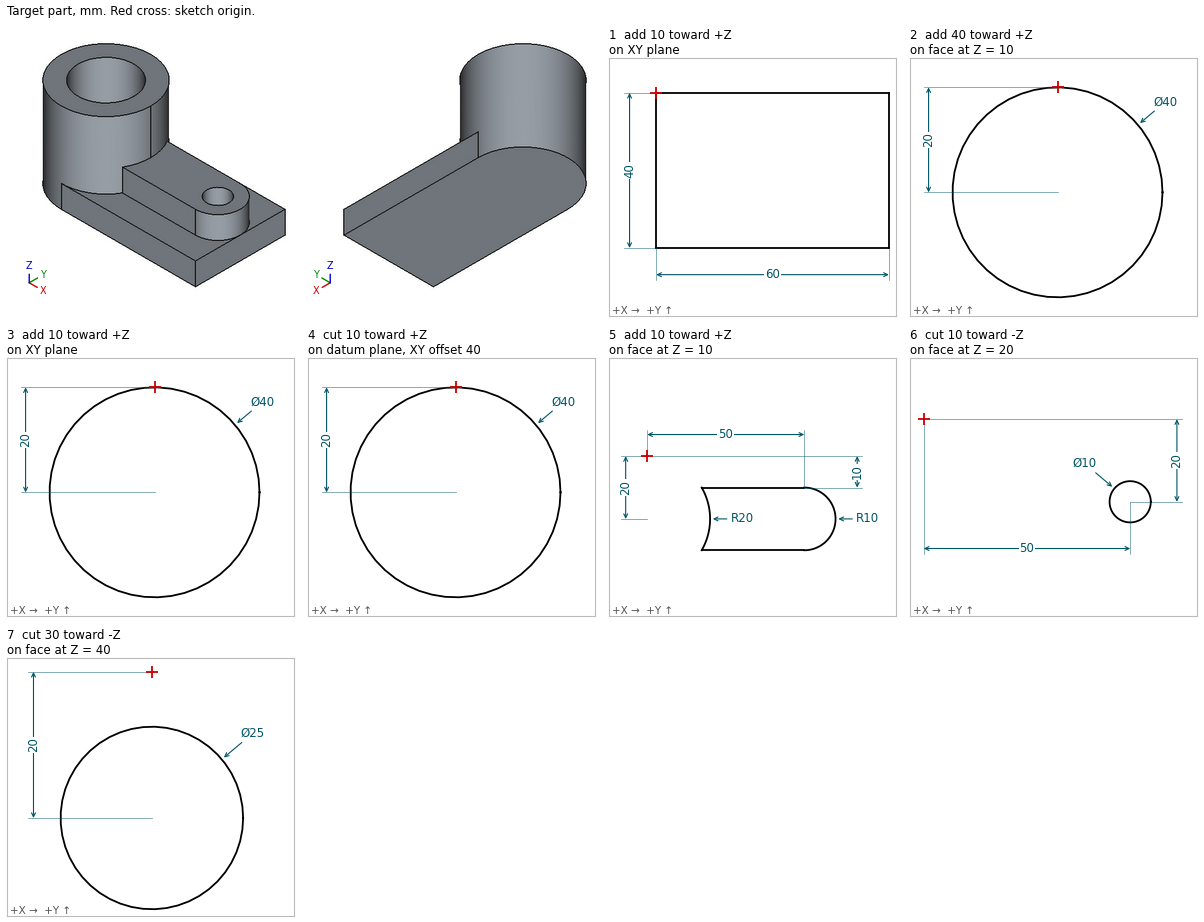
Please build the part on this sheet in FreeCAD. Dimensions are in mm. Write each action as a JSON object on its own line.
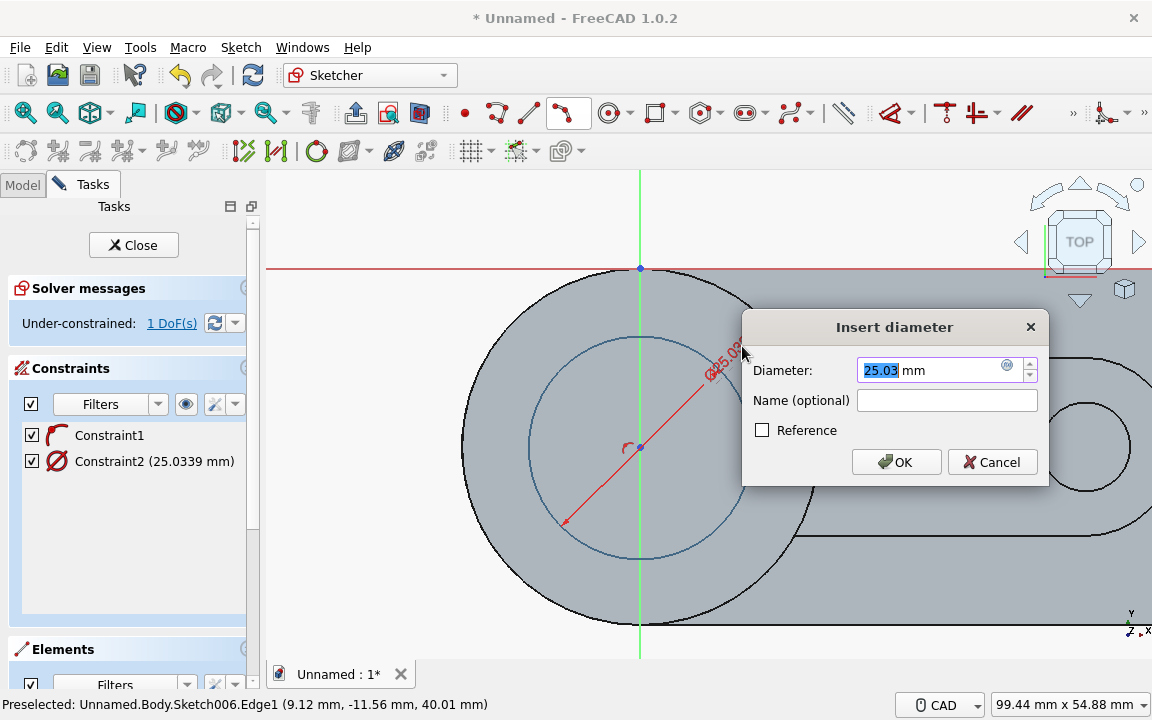
{"action": "type", "text": "25"}
{"action": "key", "text": "Return"}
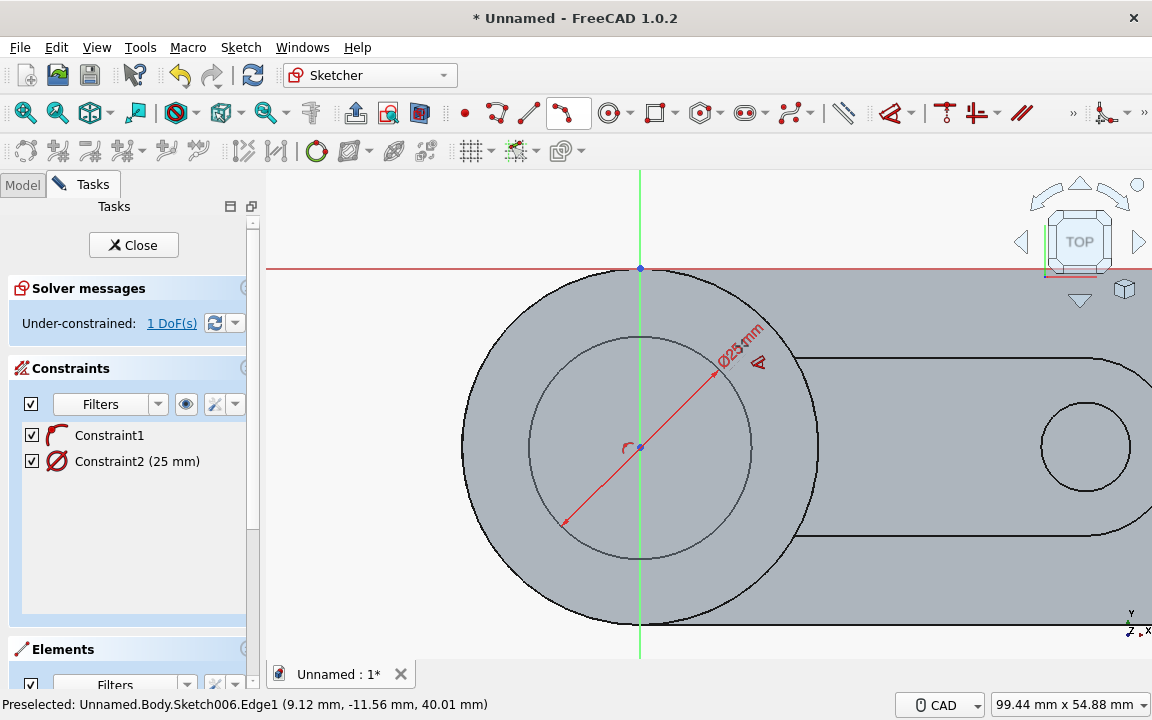
{"action": "left_click", "coordinate": [640, 448]}
{"action": "left_click", "coordinate": [674, 317]}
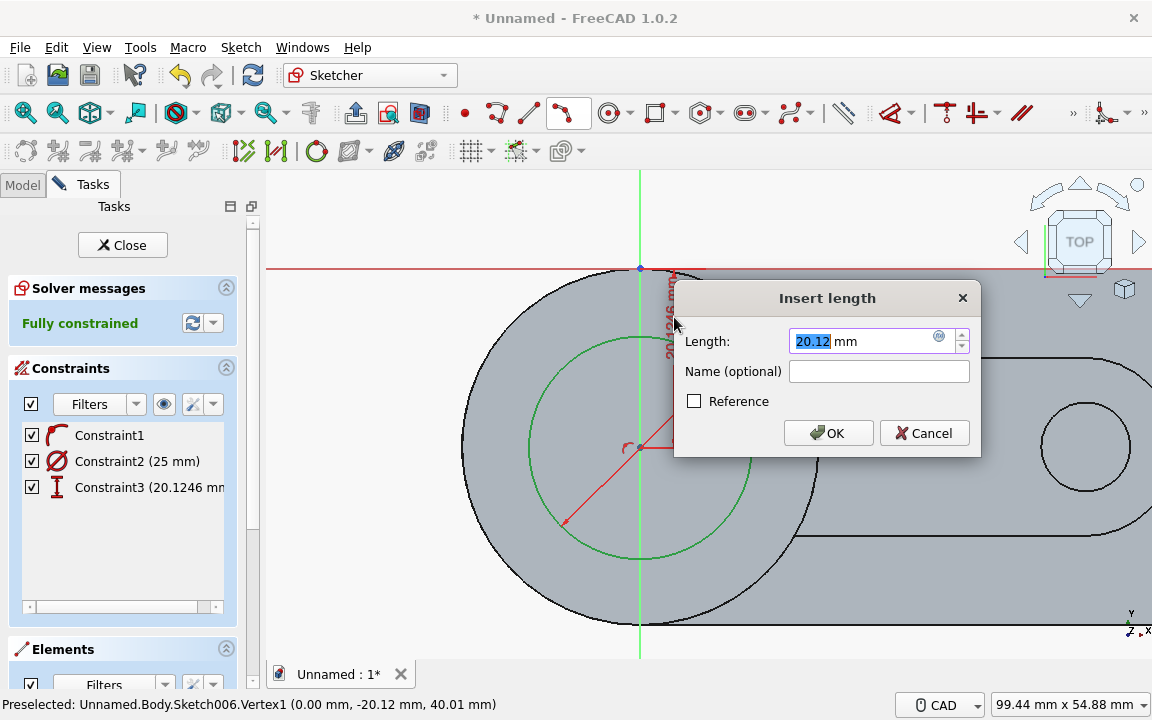
{"action": "type", "text": "20"}
{"action": "key", "text": "Return"}
{"action": "key", "text": "Escape"}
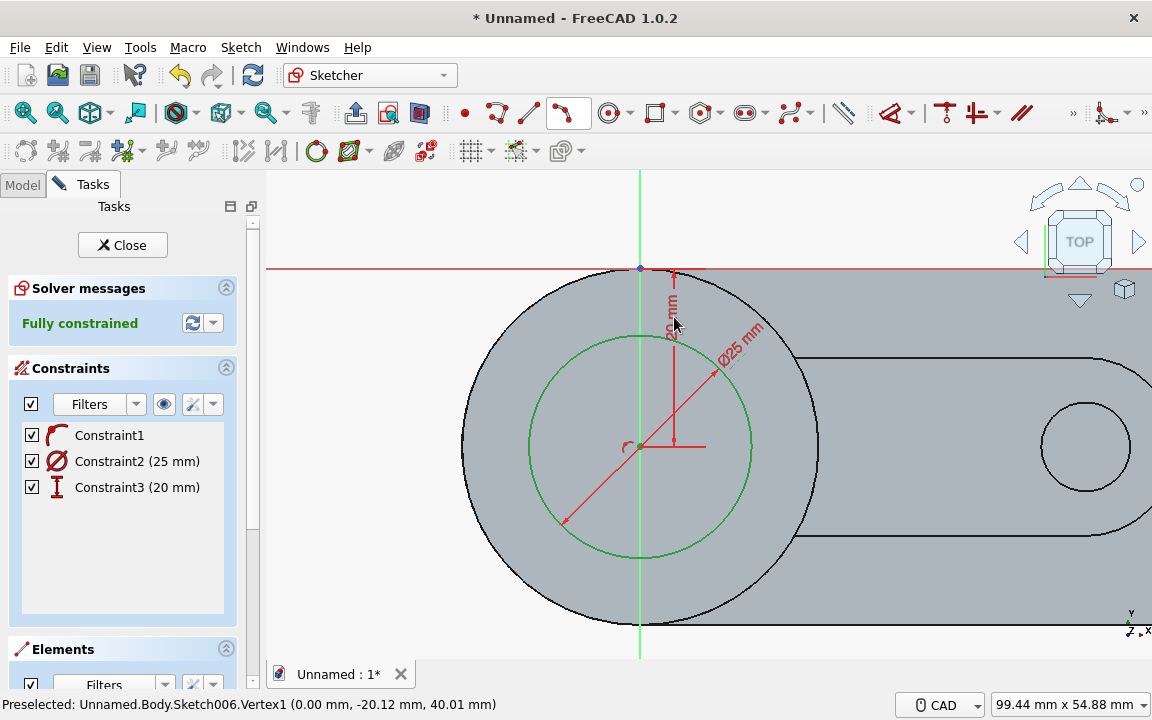
{"action": "left_click", "coordinate": [123, 245]}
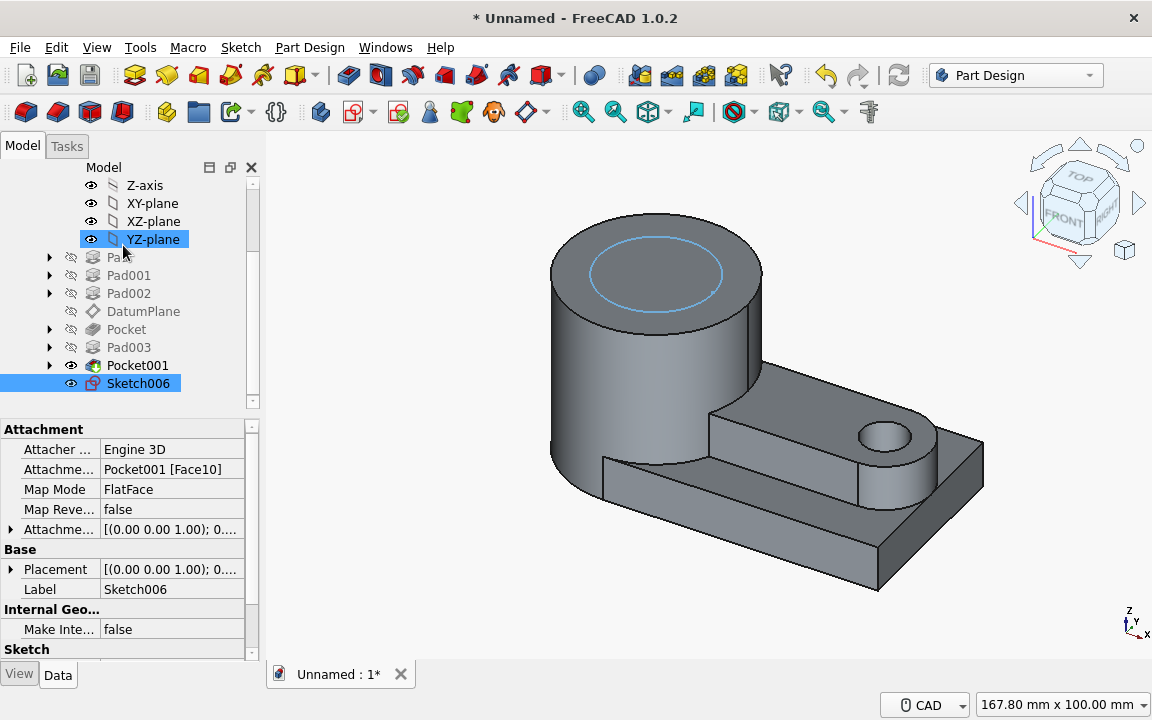
{"action": "left_click", "coordinate": [350, 76]}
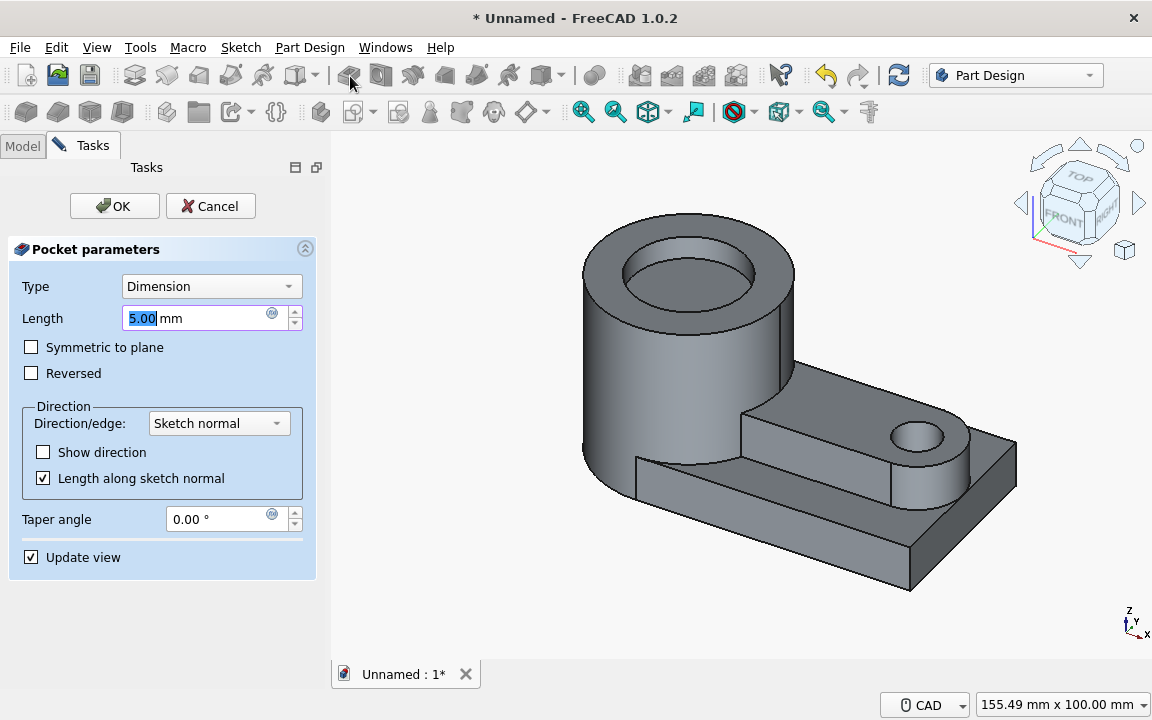
{"action": "type", "text": "30"}
{"action": "key", "text": "Tab"}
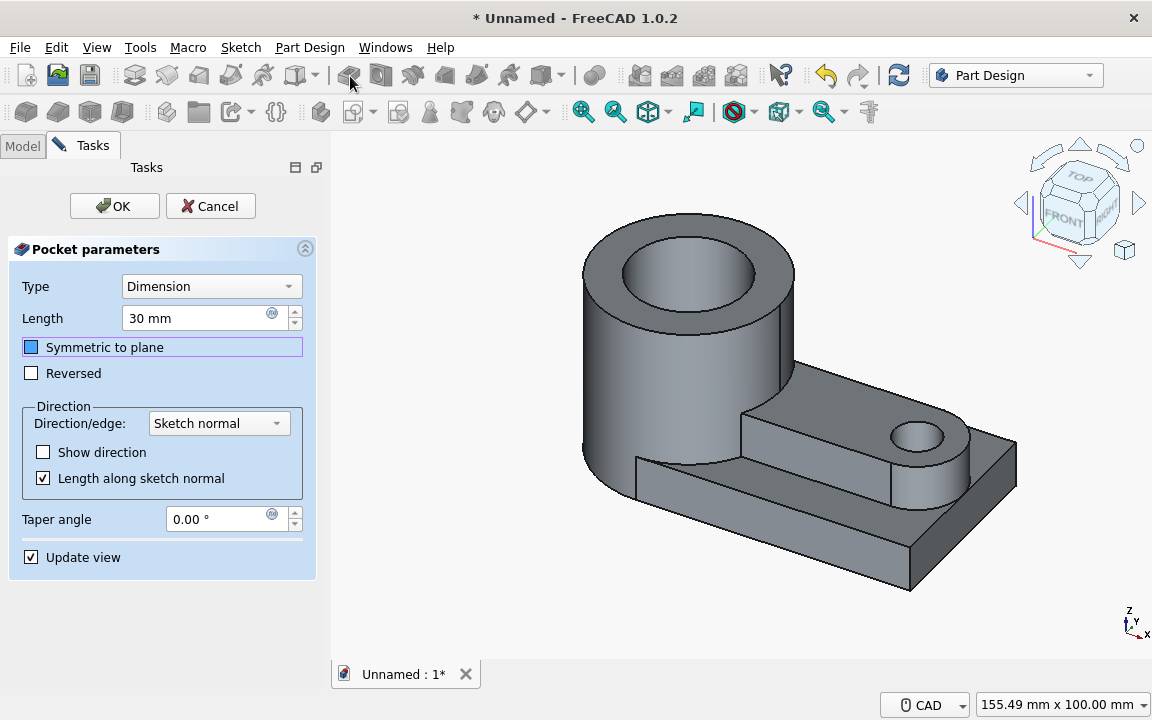
{"action": "left_click", "coordinate": [115, 206]}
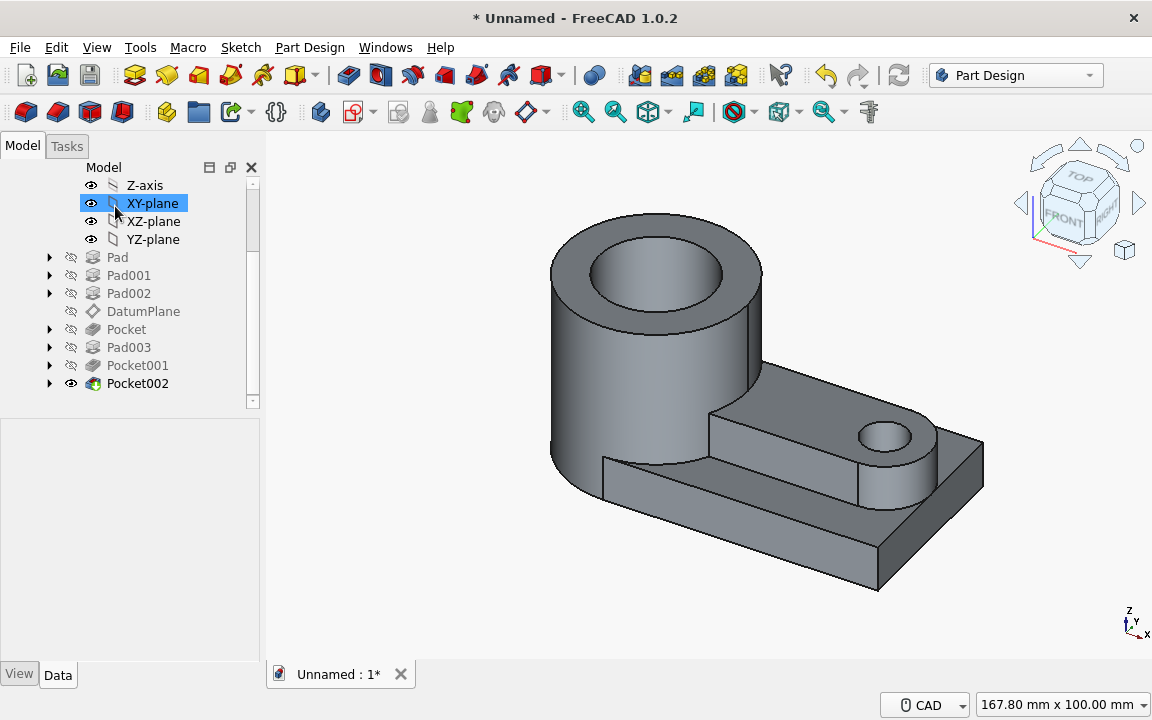
{"action": "key", "text": "0"}